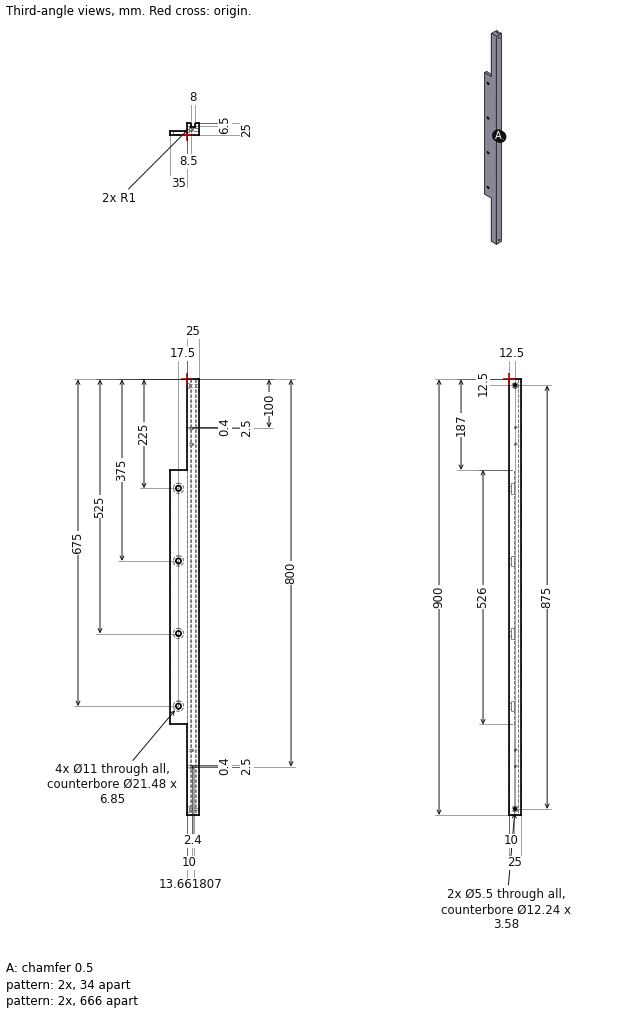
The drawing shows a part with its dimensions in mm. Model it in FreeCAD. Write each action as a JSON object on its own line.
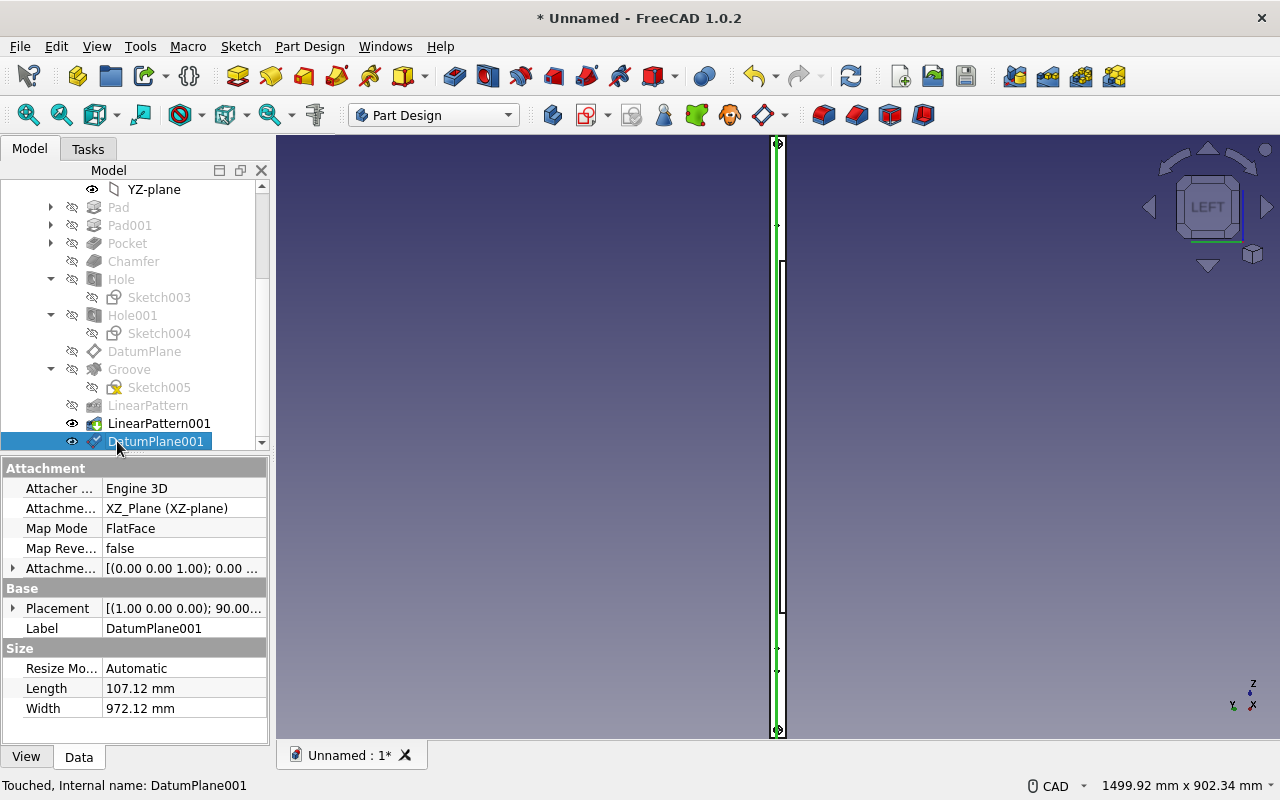
{"action": "left_click", "coordinate": [586, 116]}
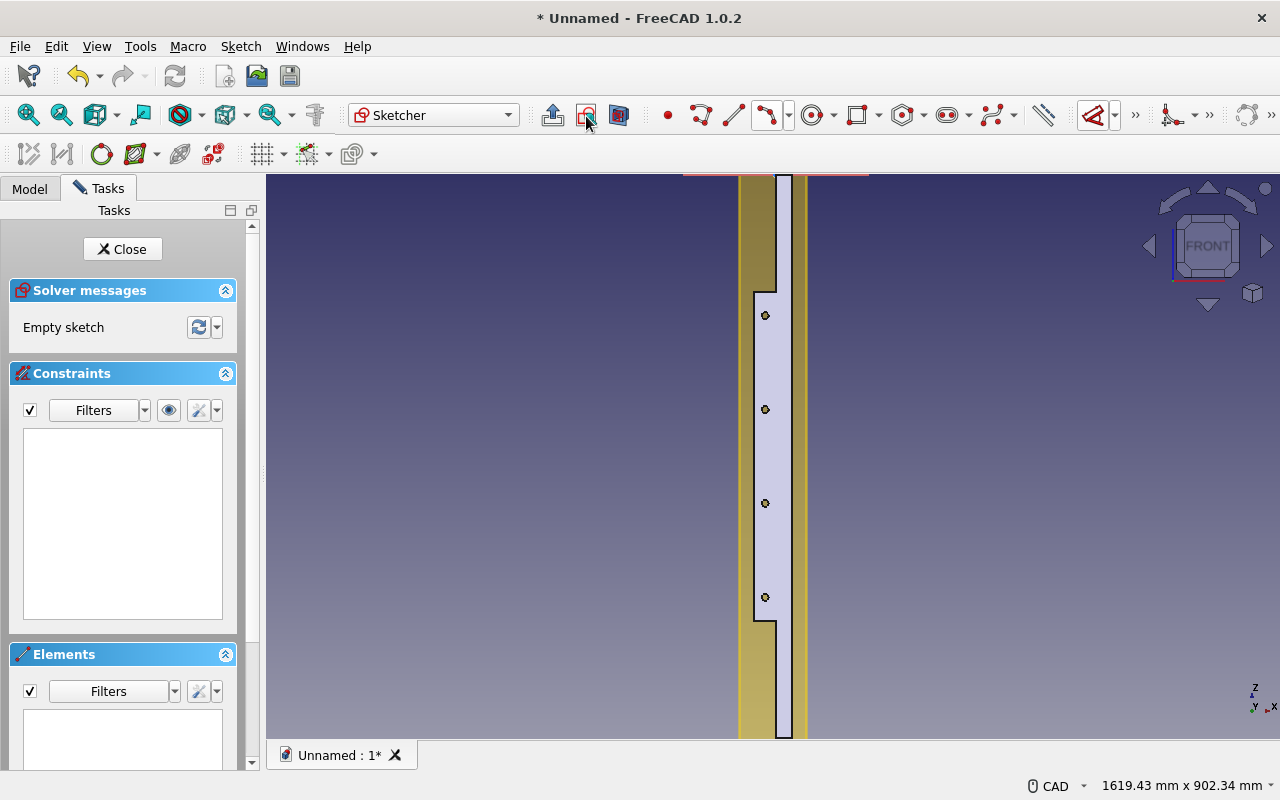
{"action": "left_click", "coordinate": [619, 116]}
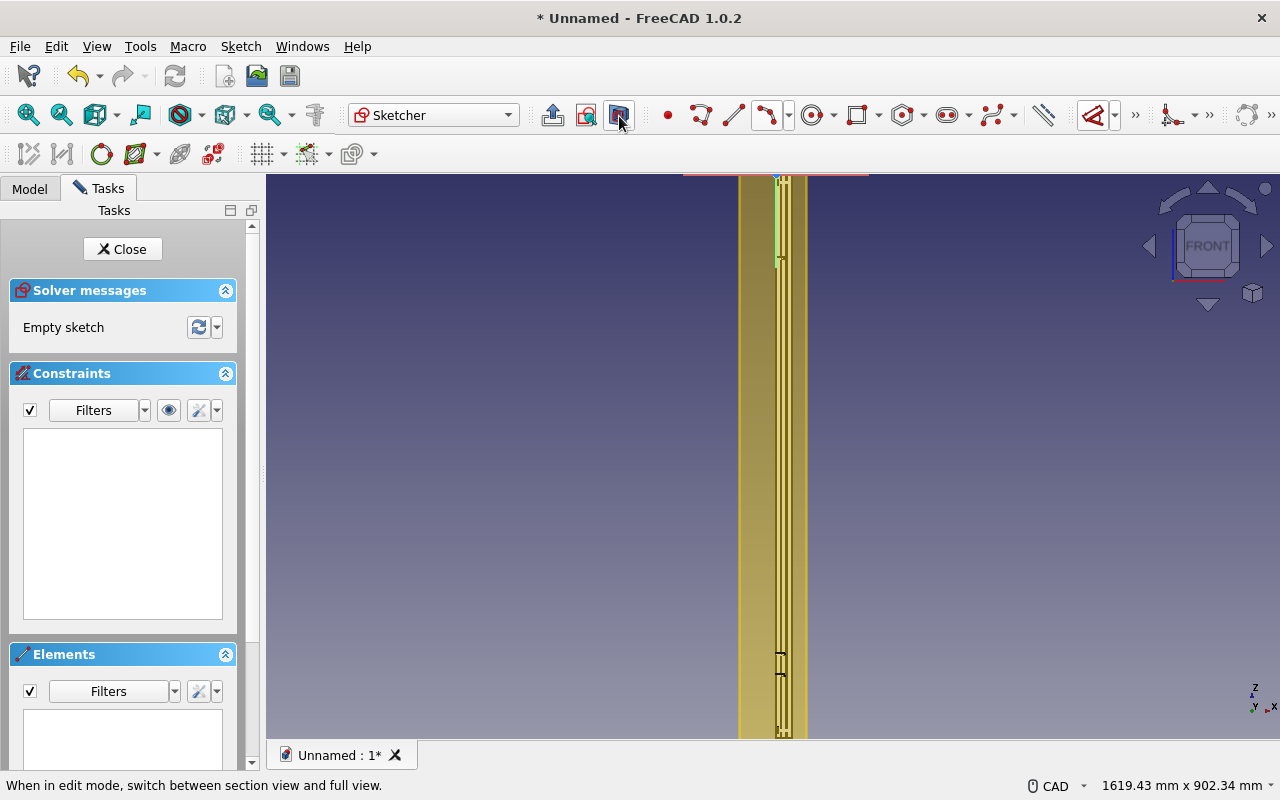
{"action": "scroll", "coordinate": [786, 225], "scroll_direction": "up", "scroll_amount": 15}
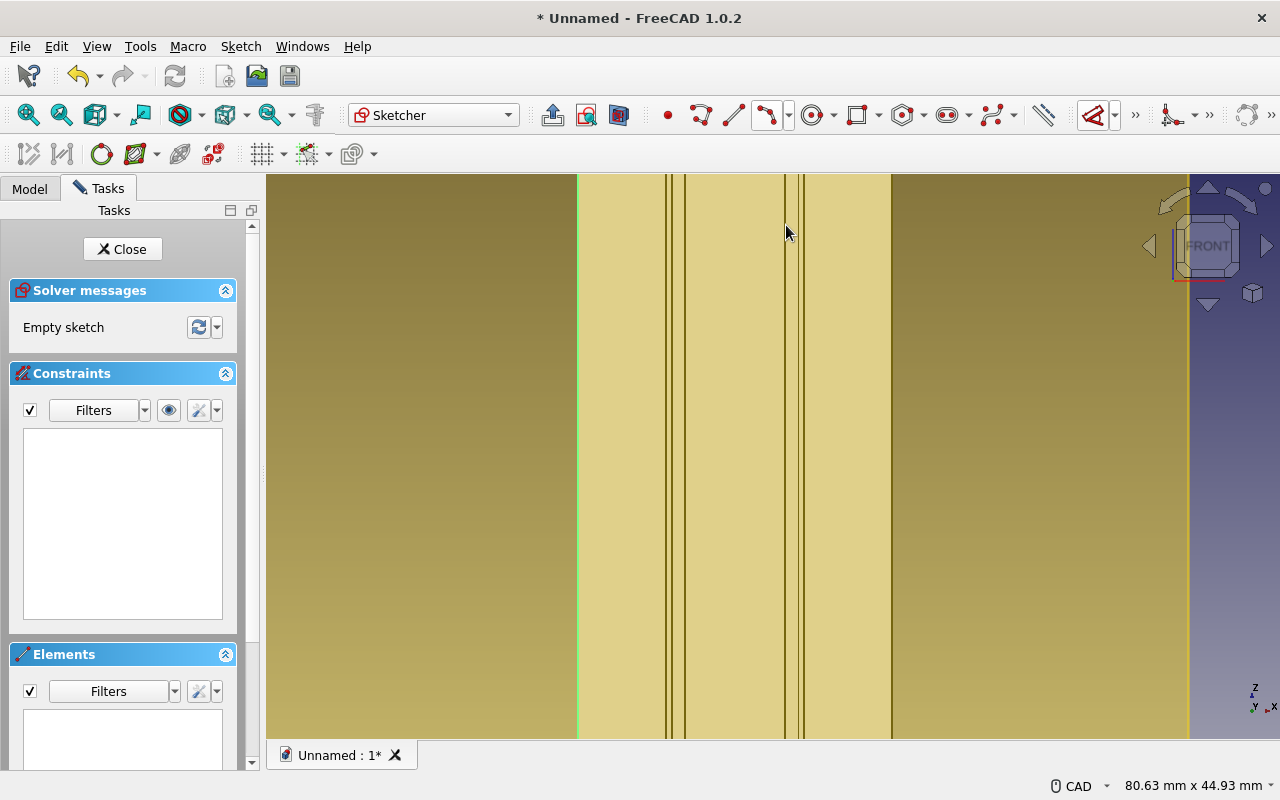
{"action": "scroll", "coordinate": [693, 455], "scroll_direction": "up", "scroll_amount": 4}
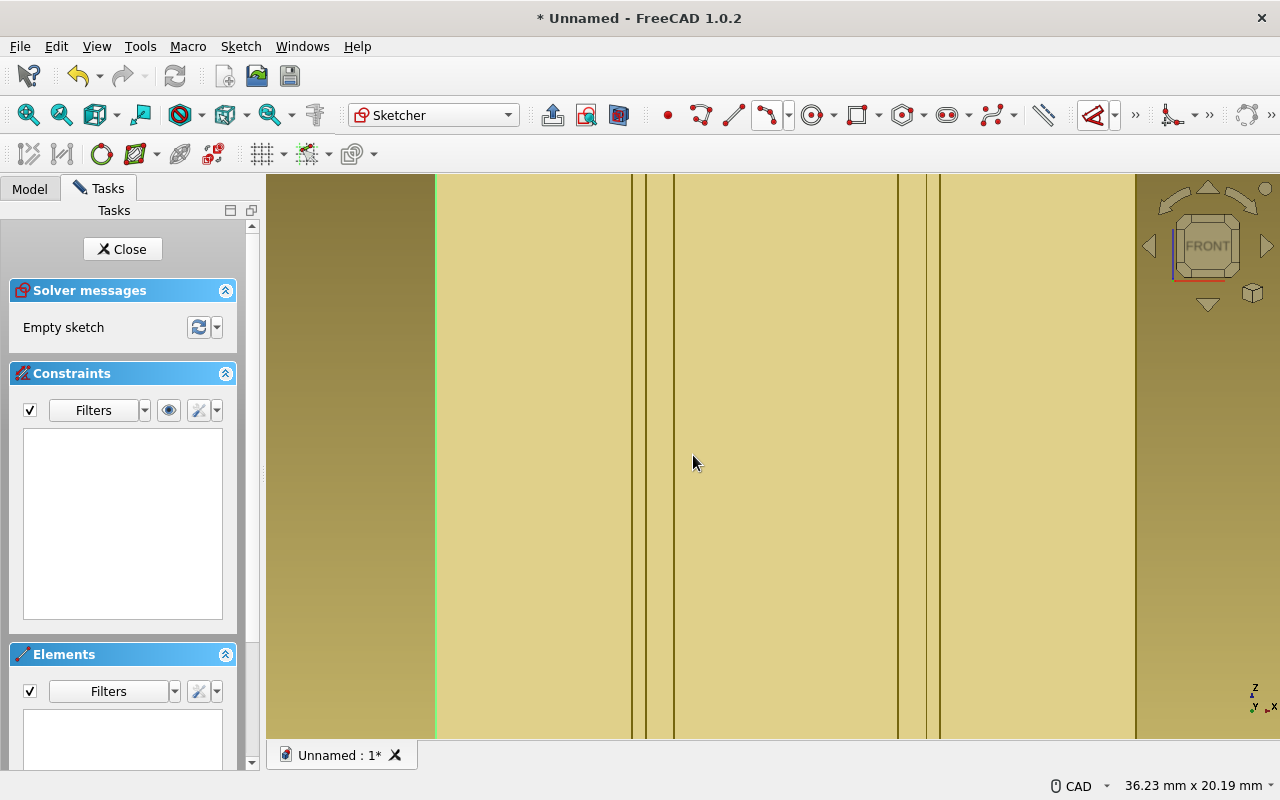
{"action": "left_click", "coordinate": [701, 116]}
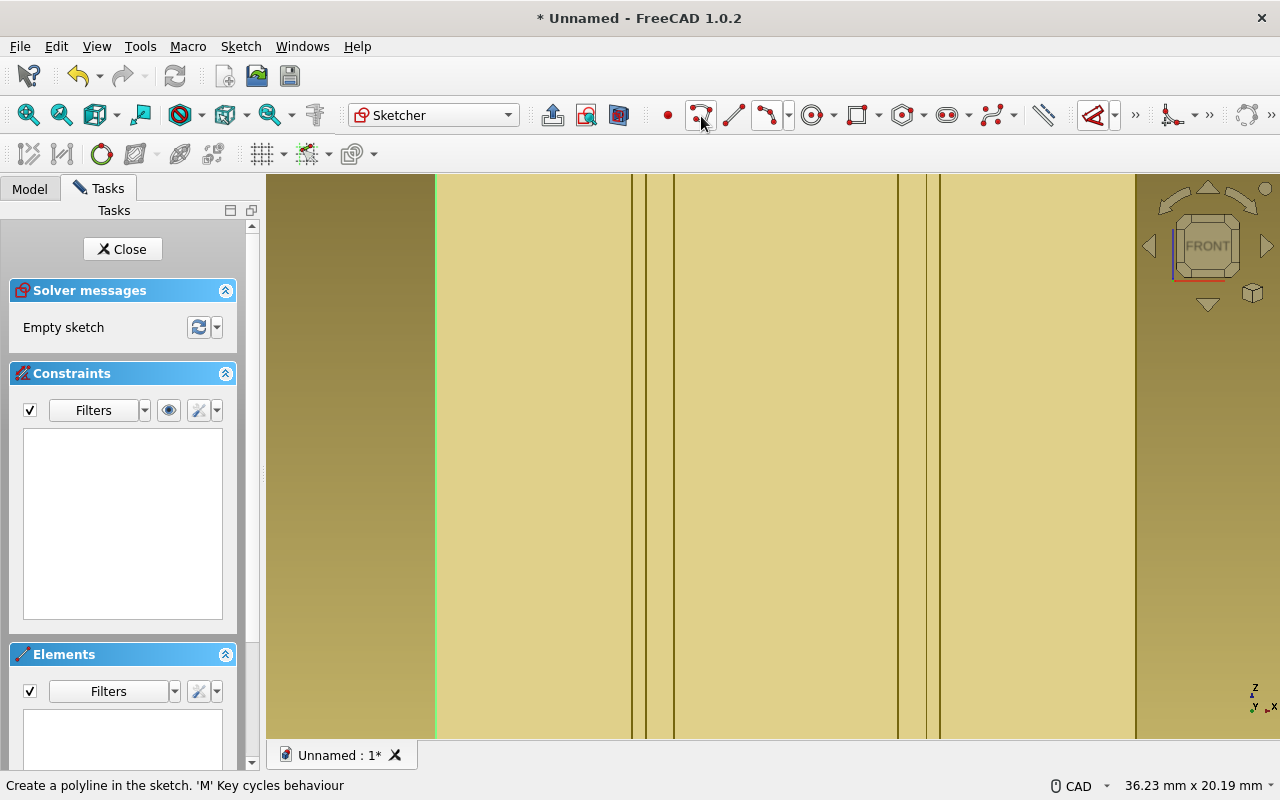
{"action": "left_click", "coordinate": [436, 421]}
{"action": "left_click", "coordinate": [716, 421]}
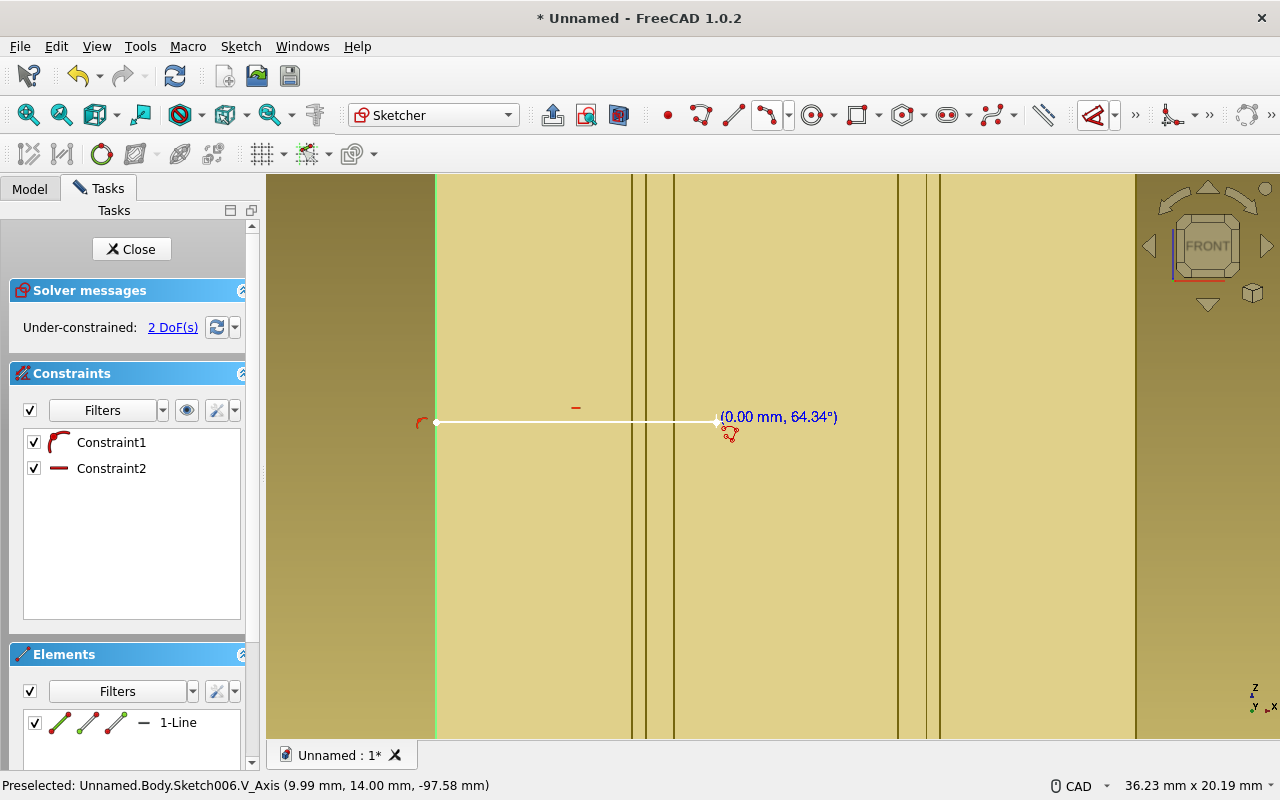
{"action": "scroll", "coordinate": [716, 432], "scroll_direction": "up", "scroll_amount": 2}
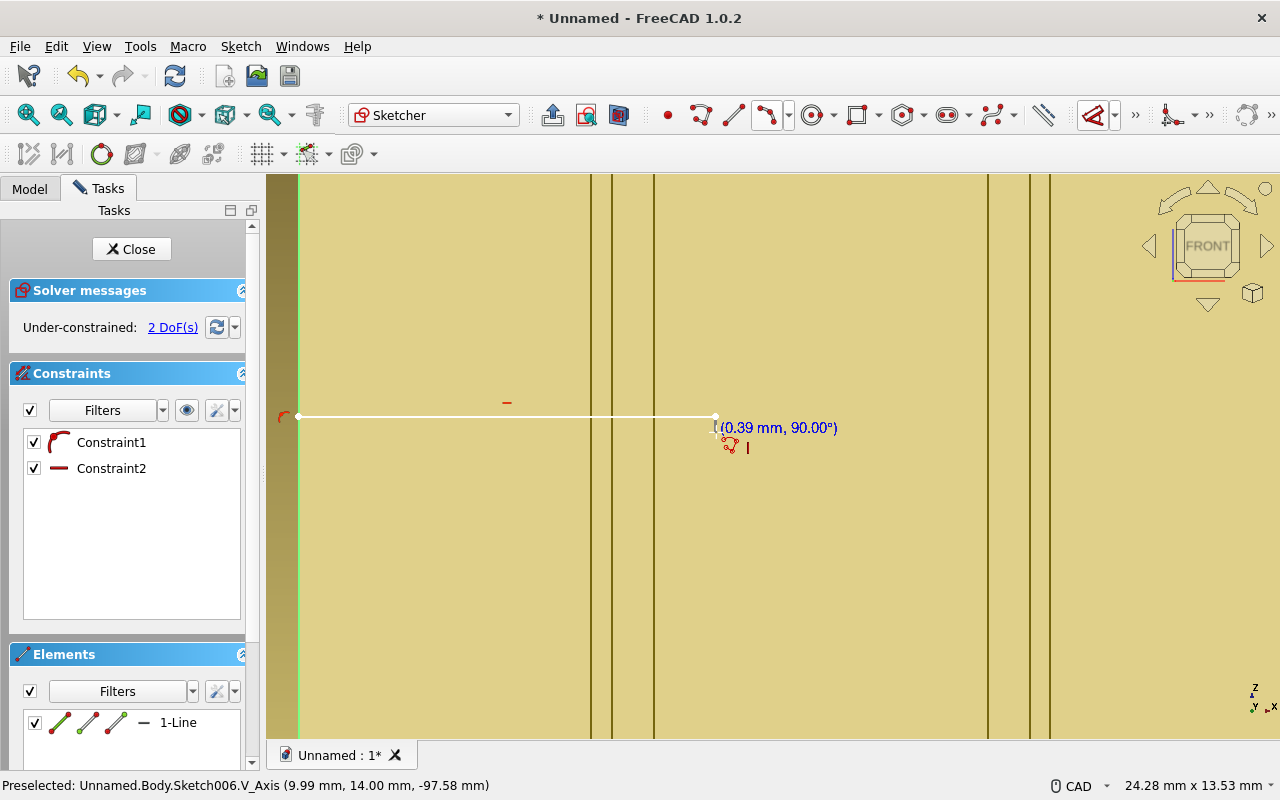
{"action": "left_click", "coordinate": [716, 432]}
{"action": "left_click", "coordinate": [817, 432]}
{"action": "left_click", "coordinate": [869, 519]}
{"action": "left_click", "coordinate": [308, 519]}
{"action": "left_click", "coordinate": [299, 417]}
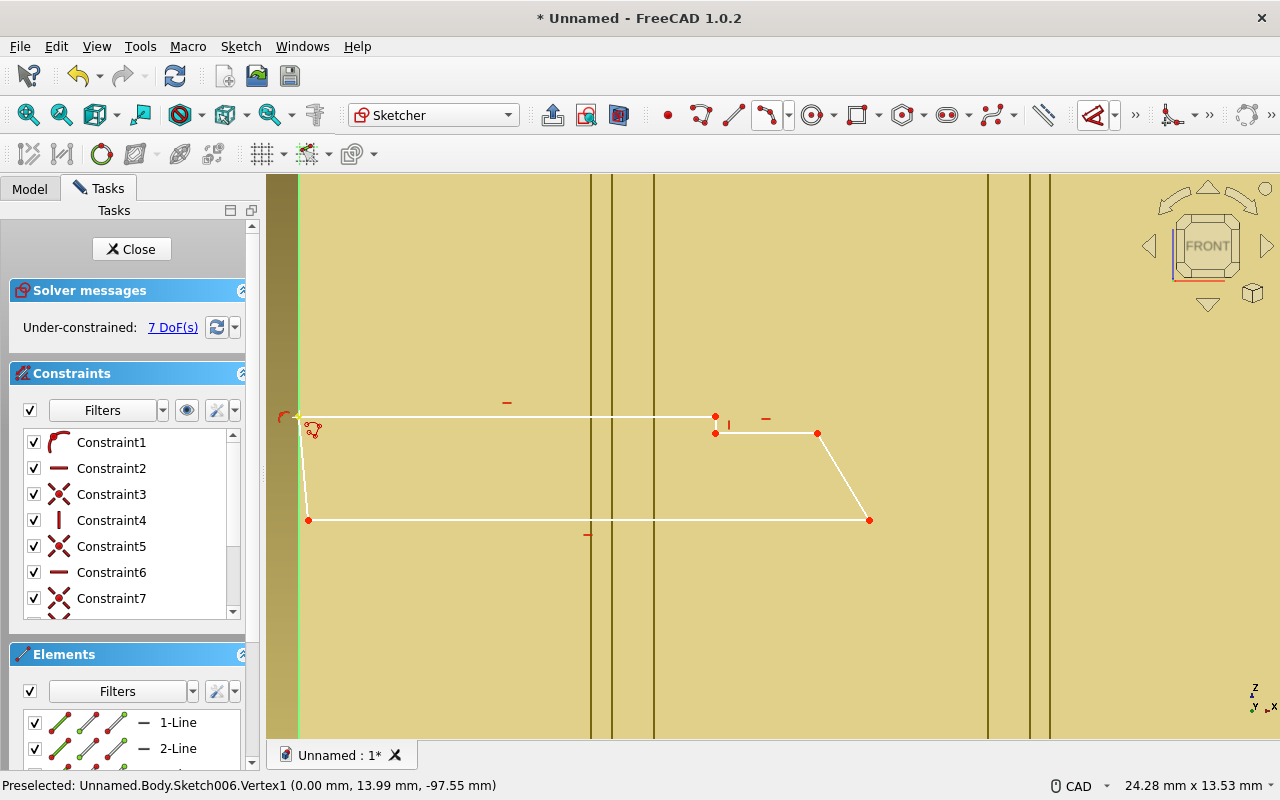
{"action": "left_click", "coordinate": [734, 116]}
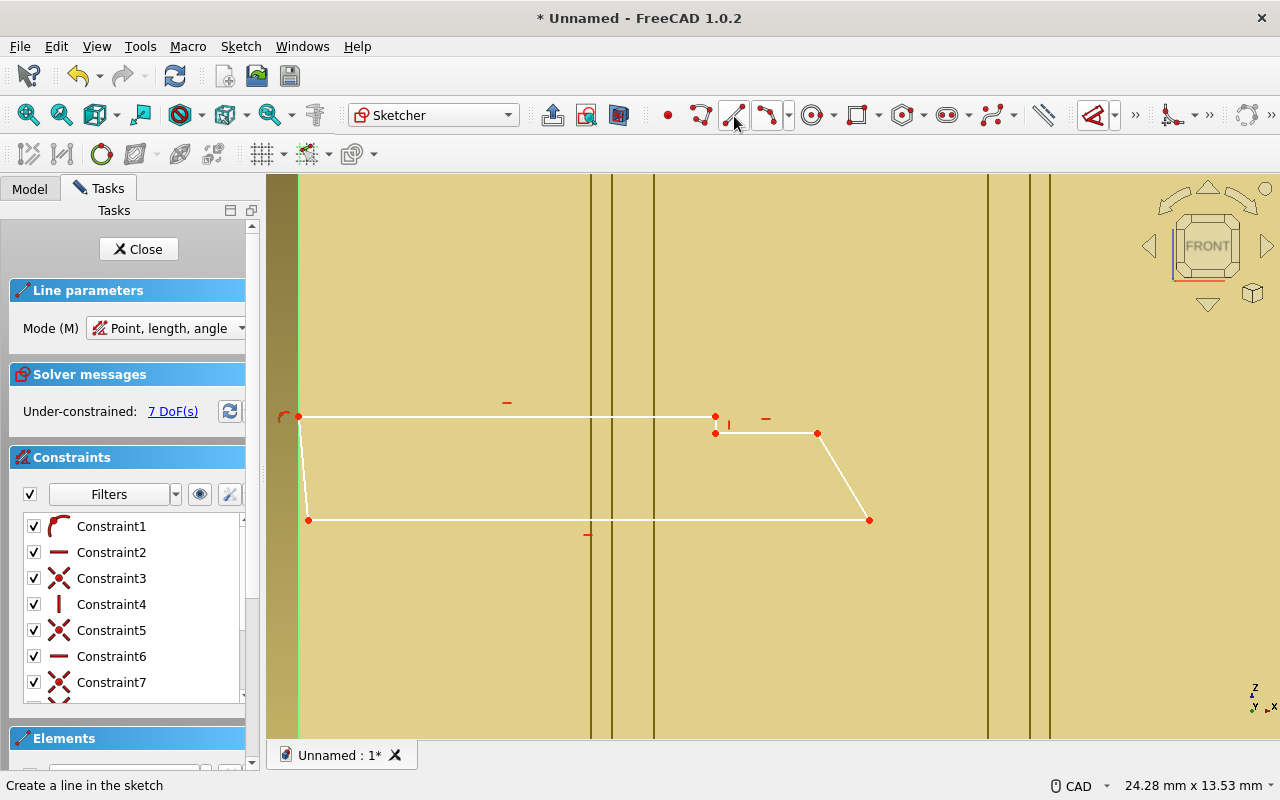
{"action": "left_click", "coordinate": [926, 519]}
{"action": "left_click", "coordinate": [1097, 519]}
{"action": "key", "text": "Escape"}